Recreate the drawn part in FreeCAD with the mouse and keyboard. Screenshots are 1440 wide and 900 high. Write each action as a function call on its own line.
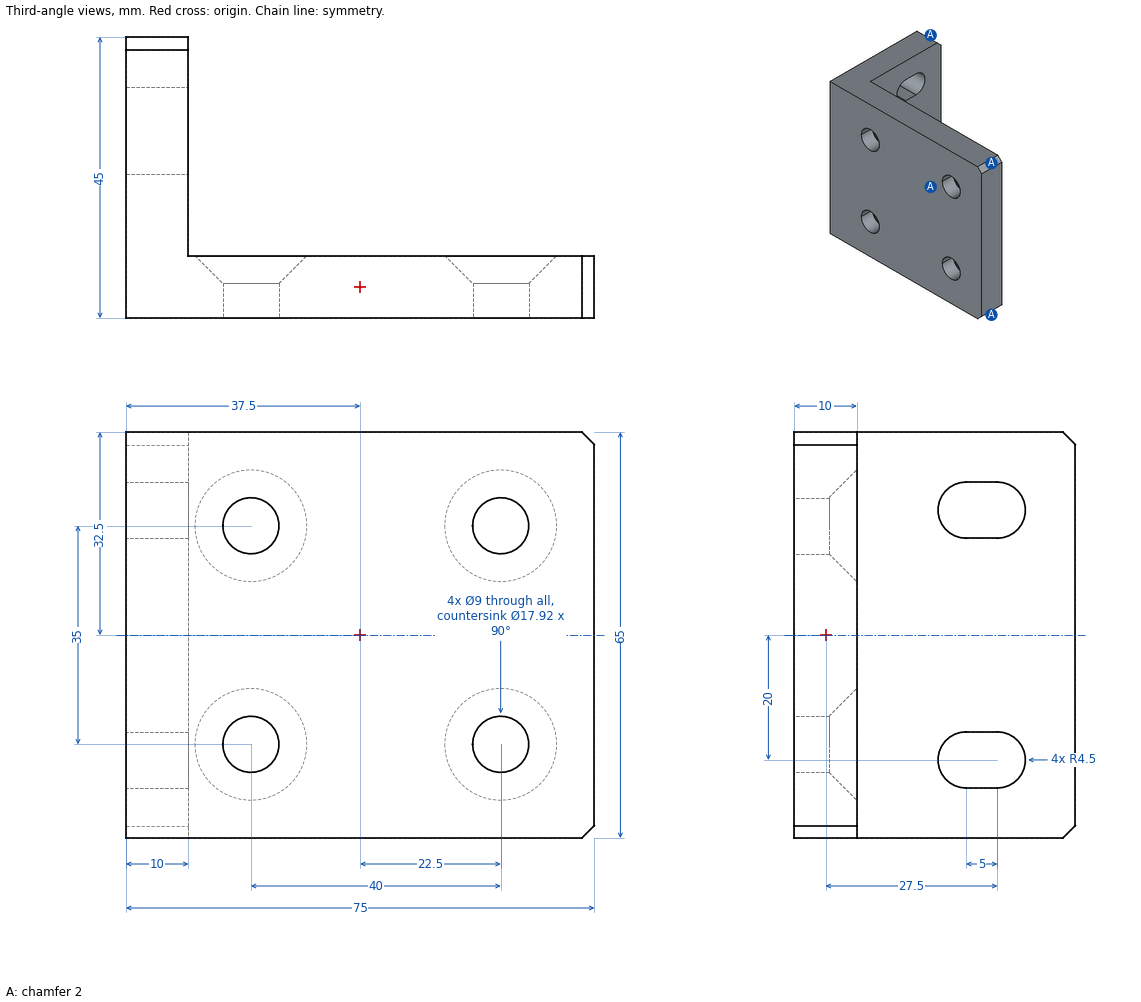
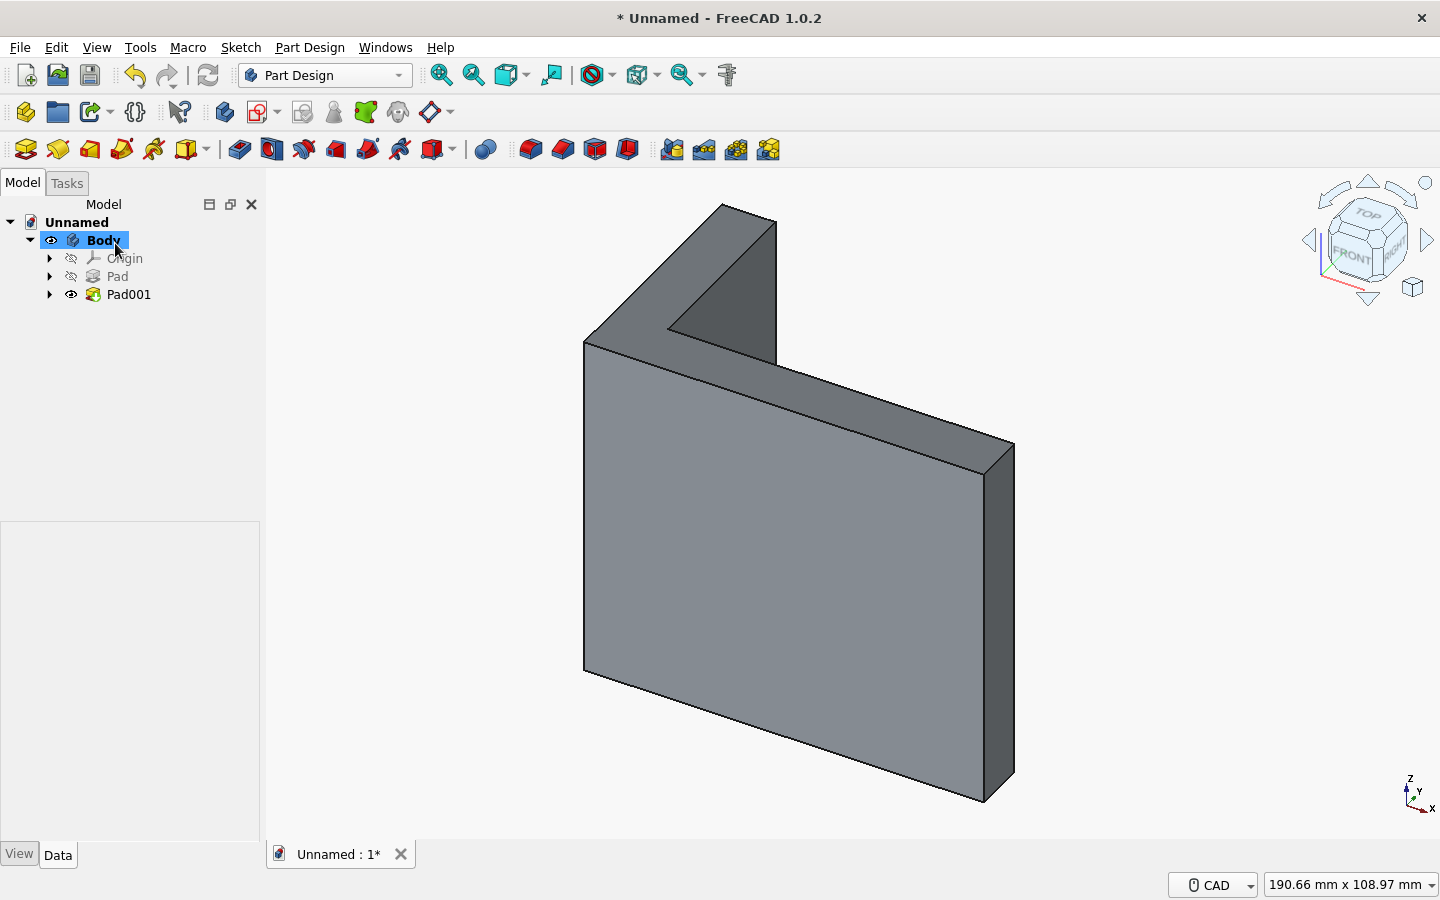
key(4)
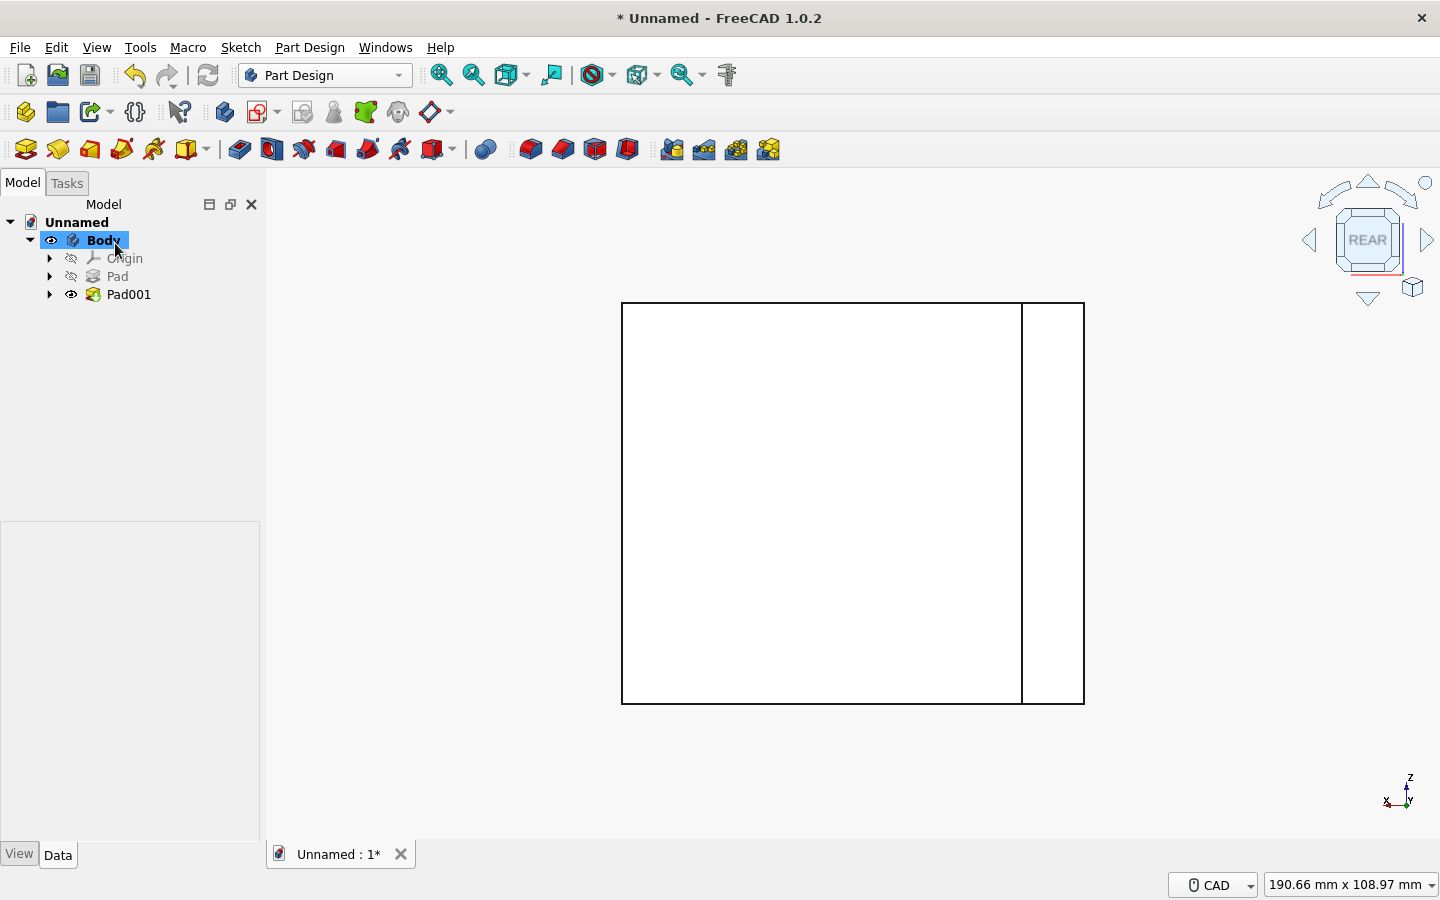
click(822, 503)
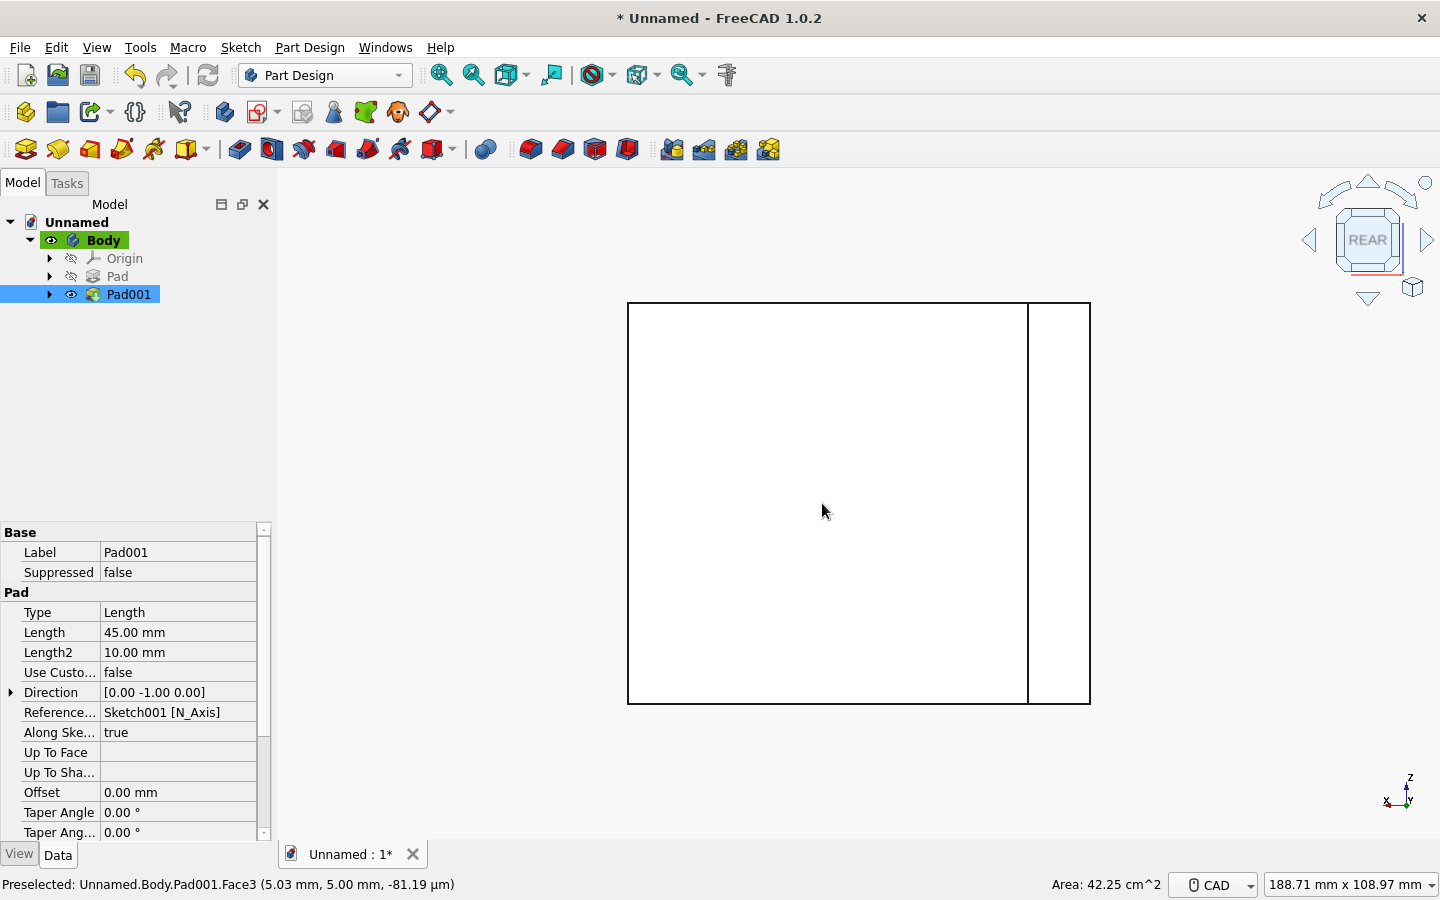
click(258, 112)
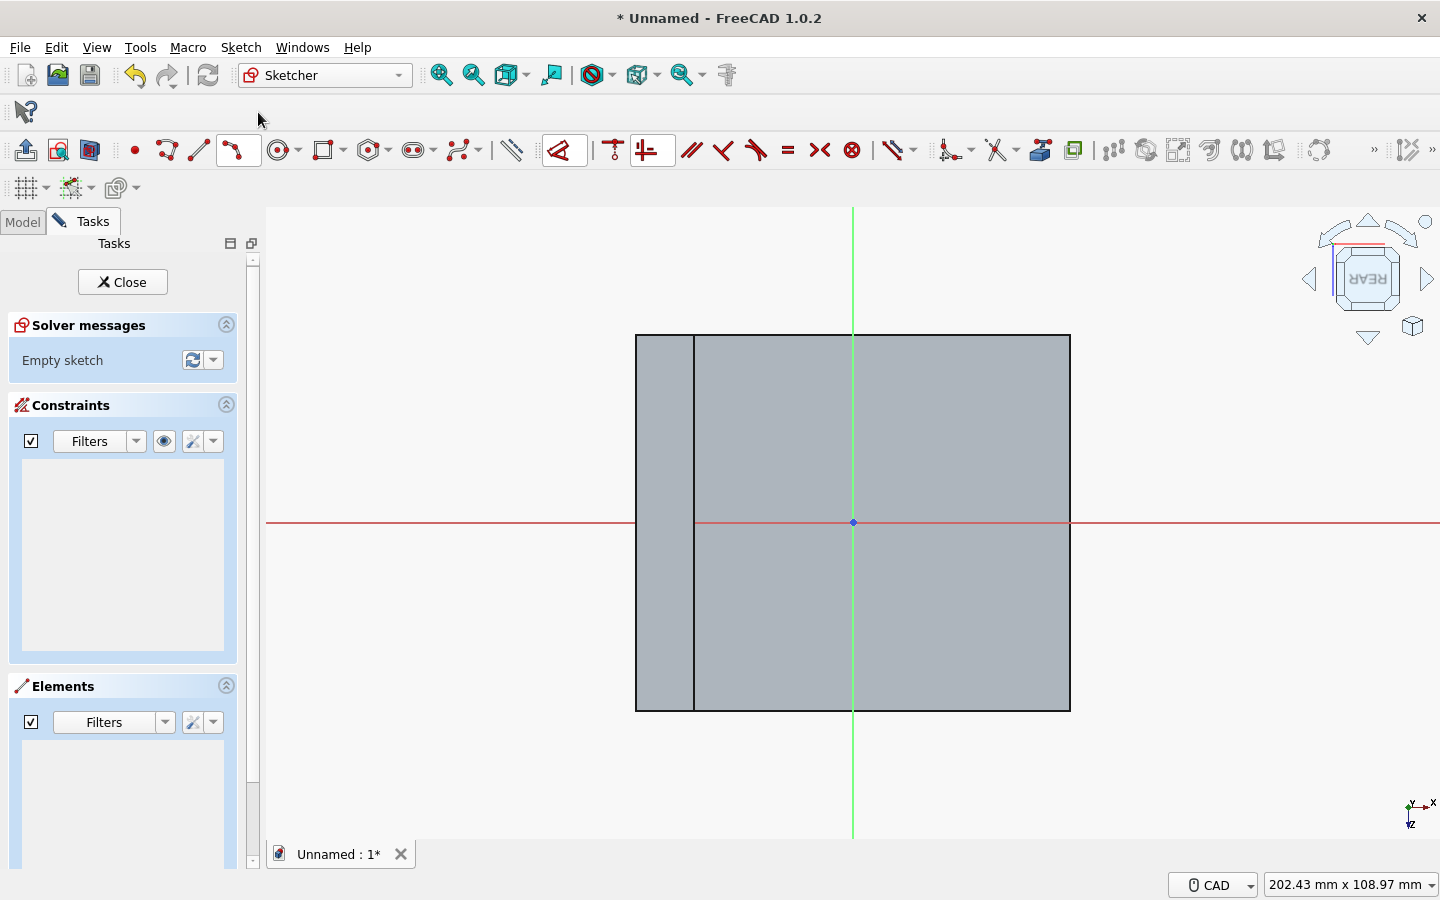
key(q)
key(s)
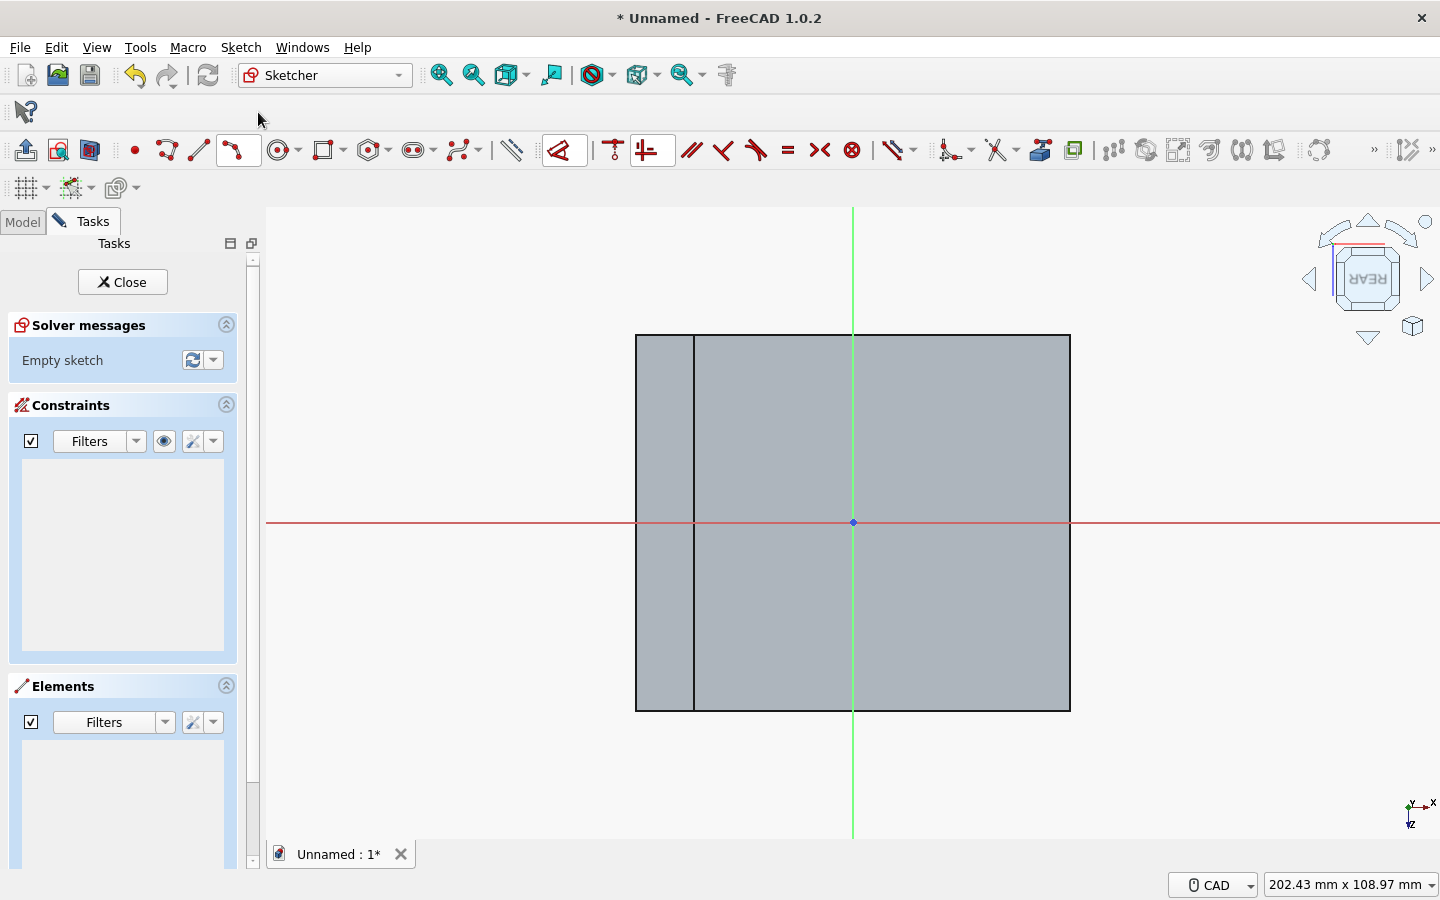
scroll(1036, 523, up, 2)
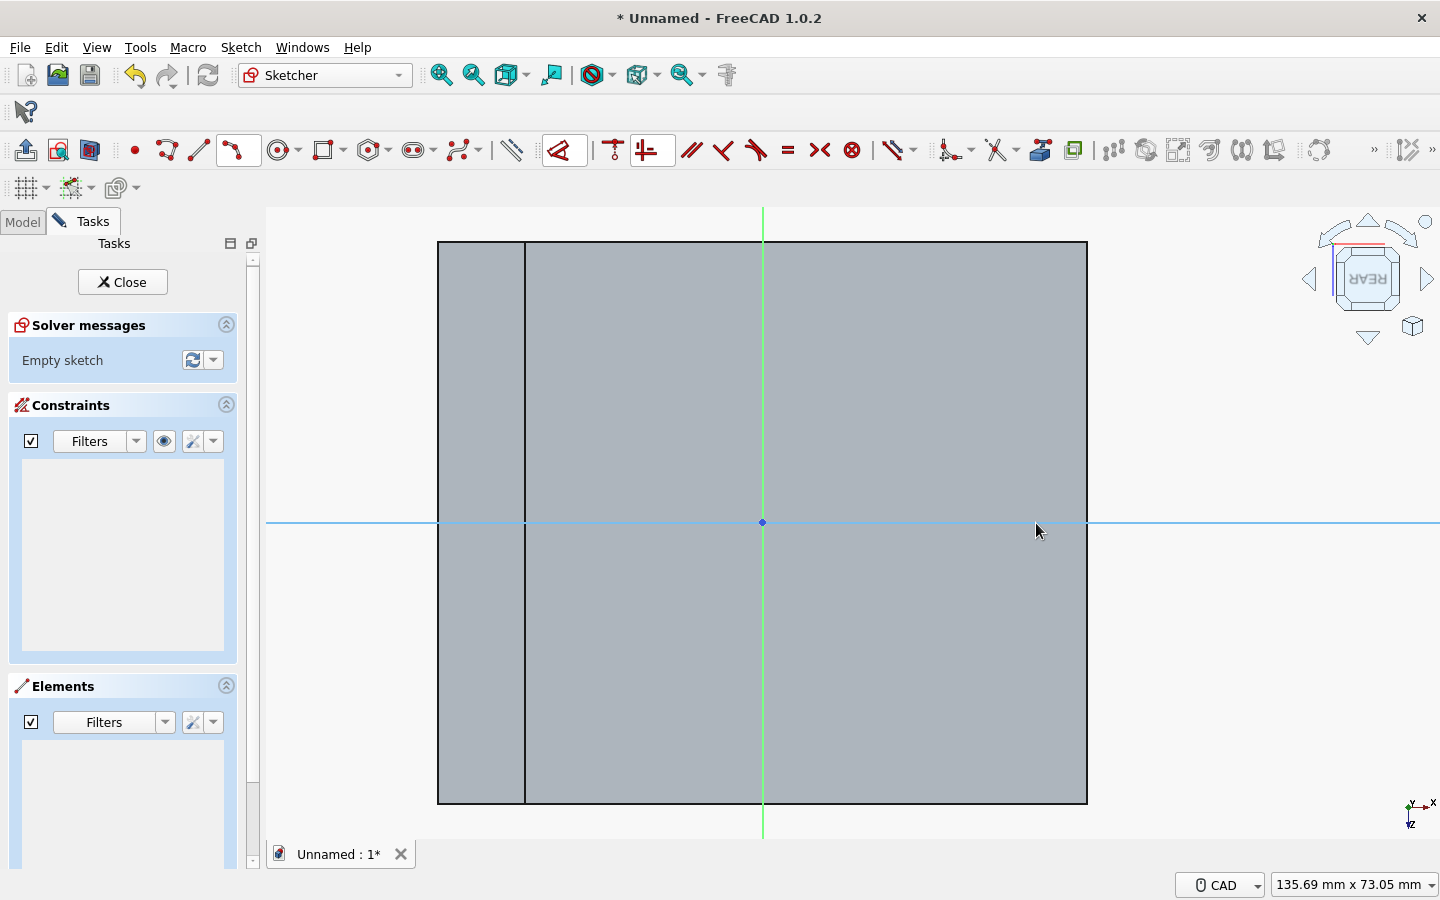
click(278, 150)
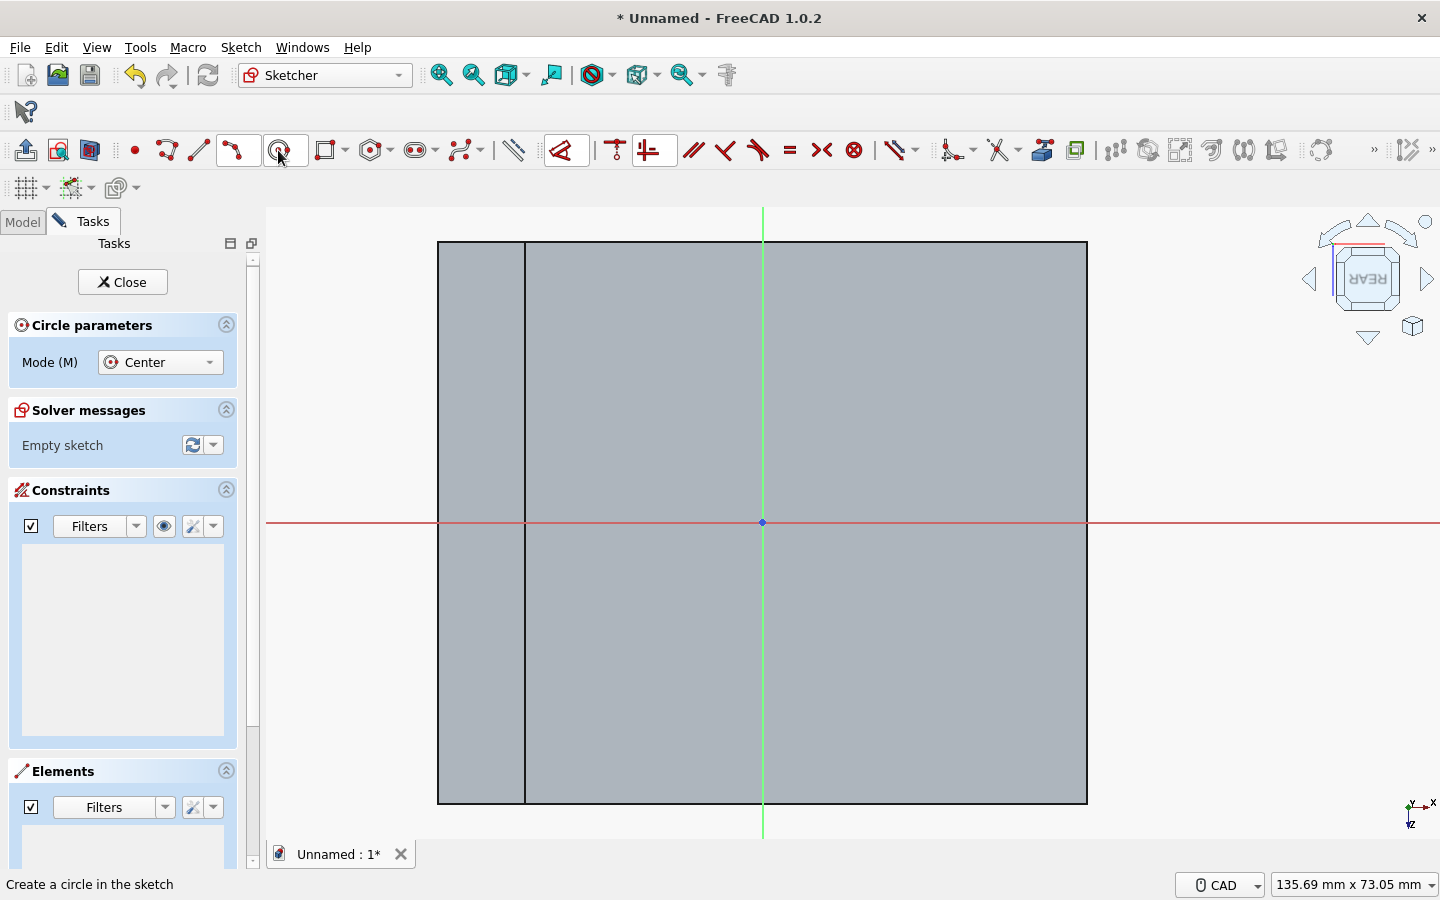
click(957, 371)
move(985, 344)